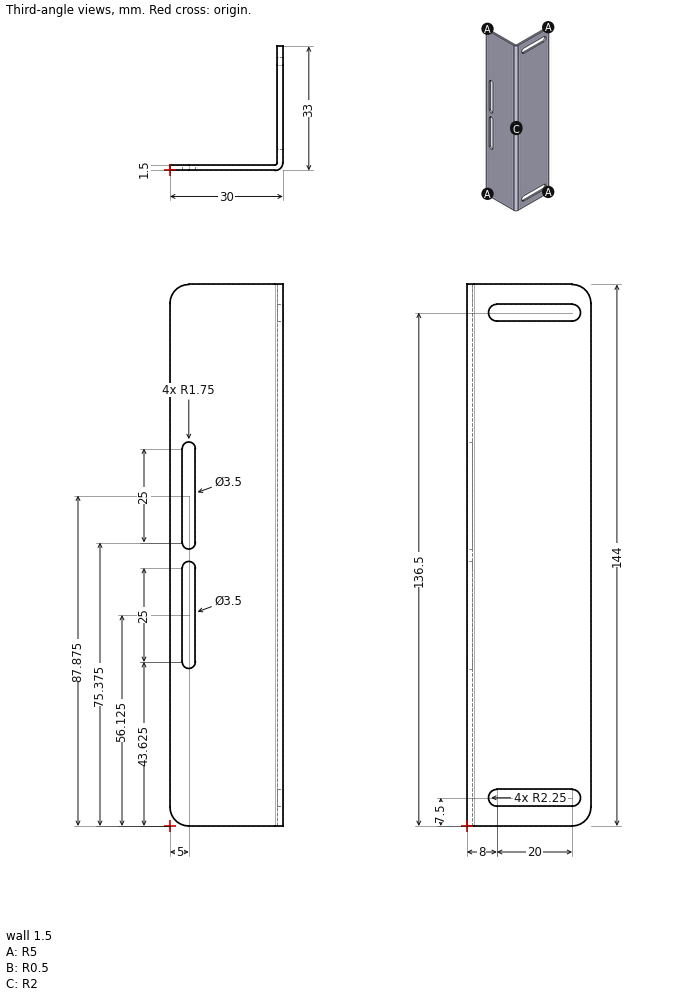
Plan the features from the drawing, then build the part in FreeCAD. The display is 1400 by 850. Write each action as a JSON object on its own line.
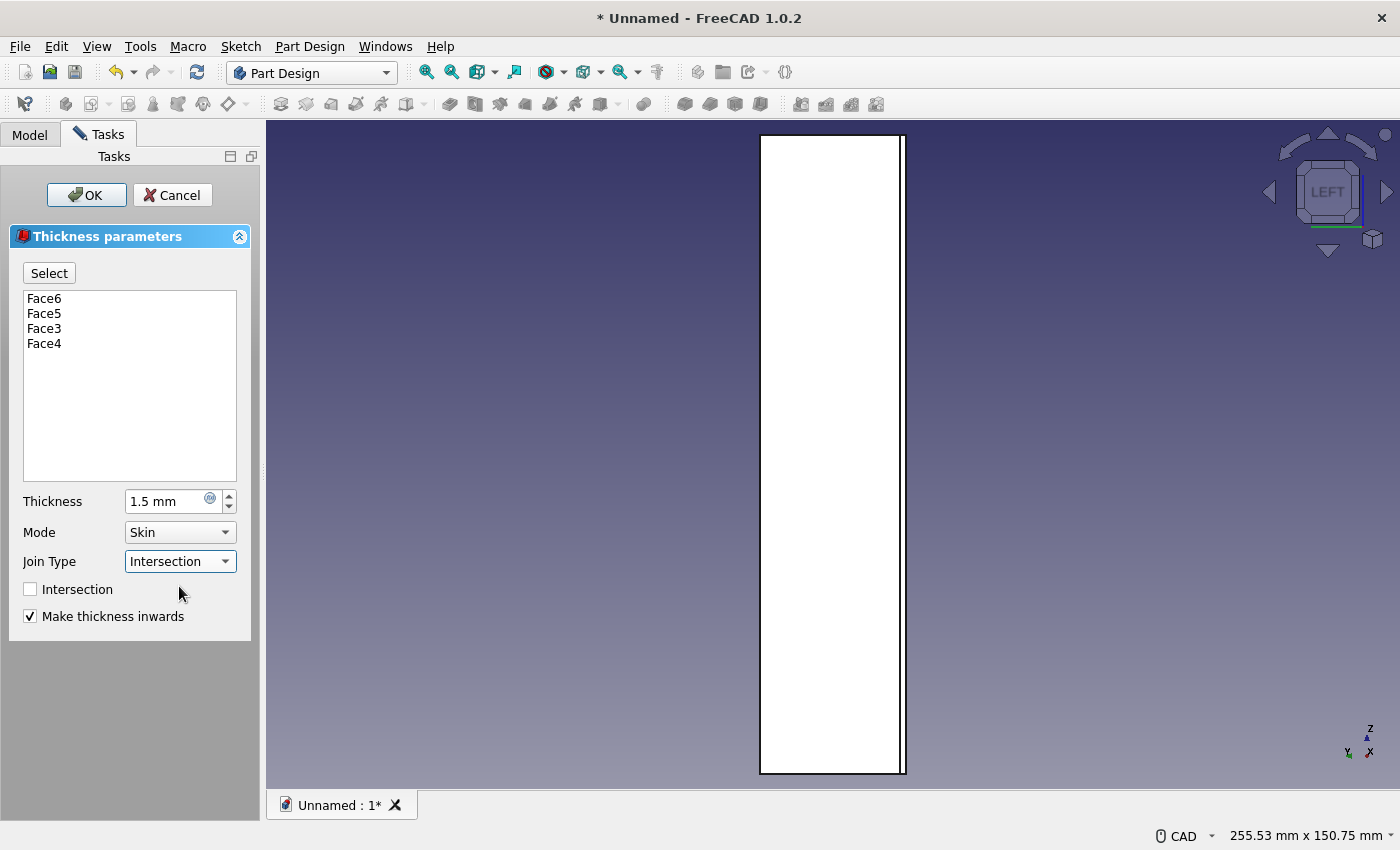
{"action": "left_click", "coordinate": [87, 195]}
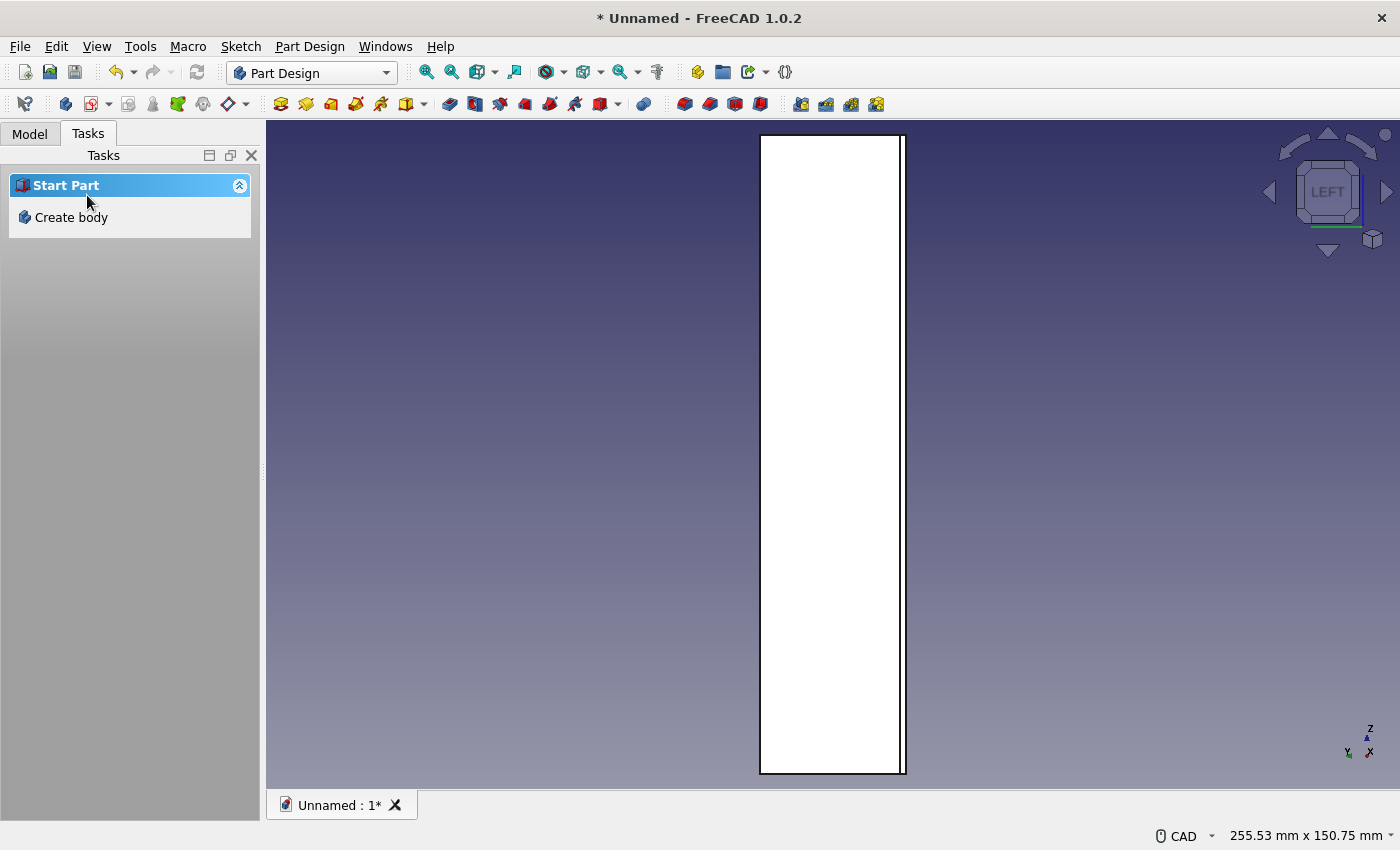
{"action": "key", "text": "0"}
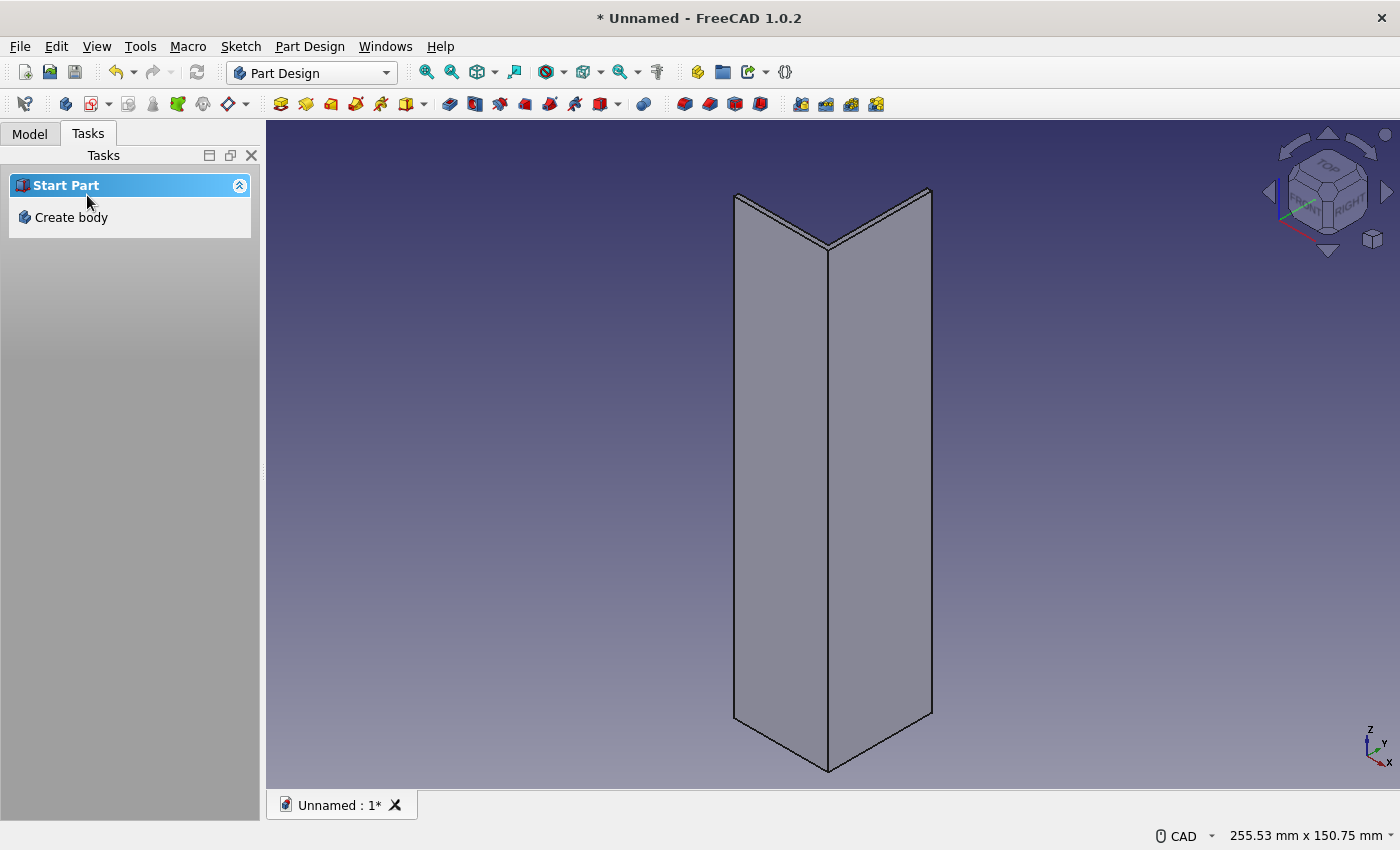
{"action": "scroll", "coordinate": [929, 189], "scroll_direction": "up", "scroll_amount": 9}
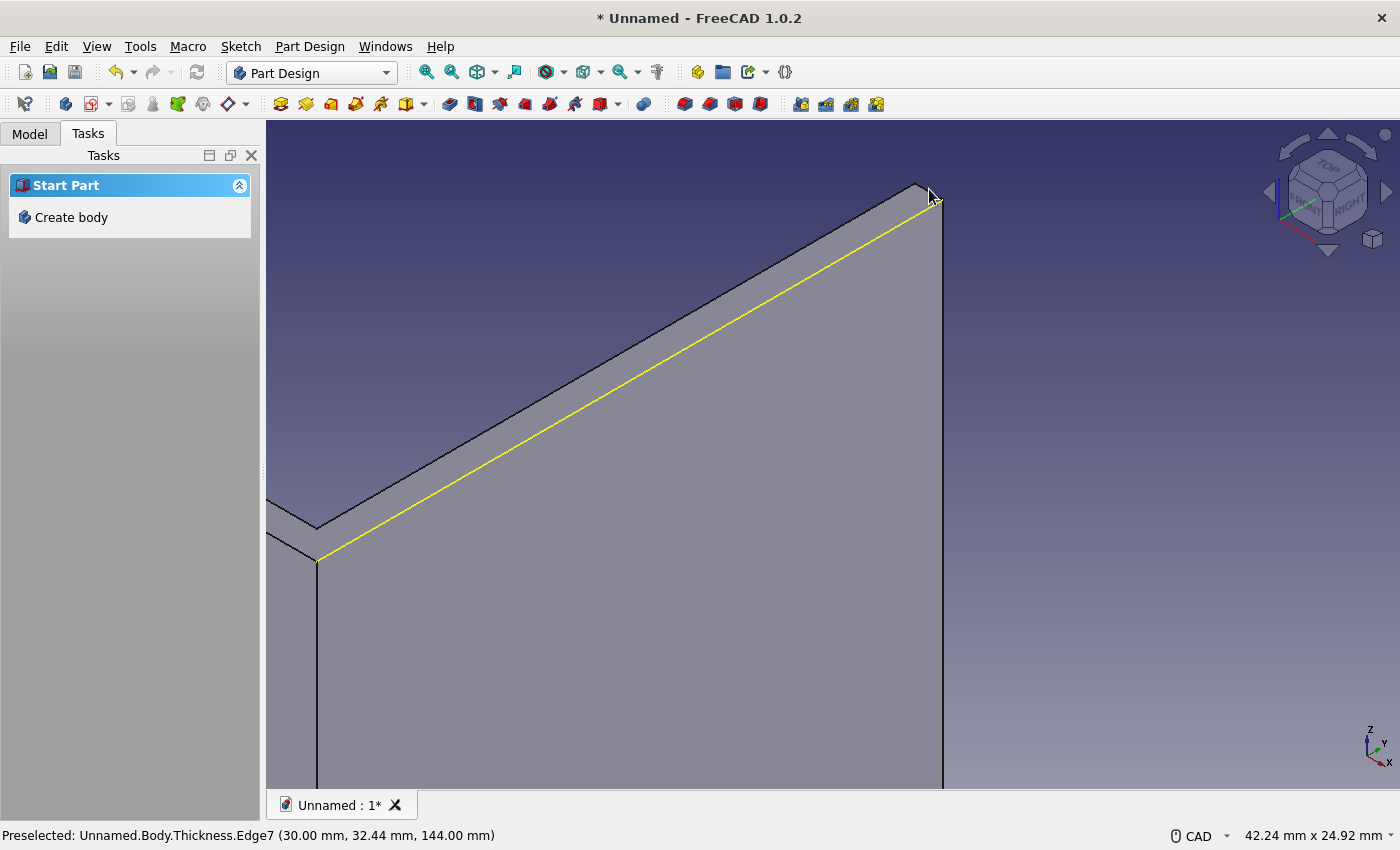
{"action": "left_click", "coordinate": [427, 72]}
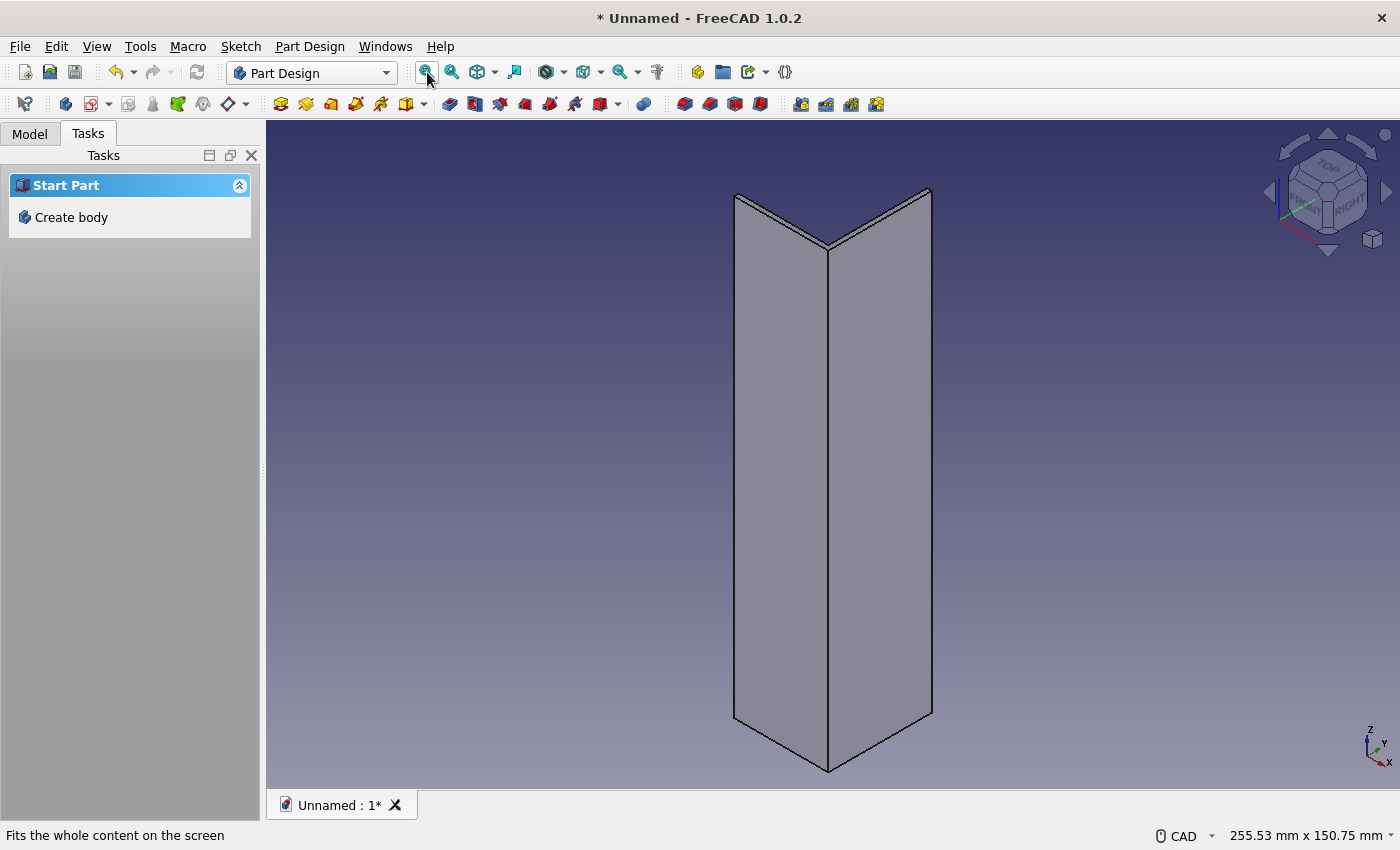
{"action": "key", "text": "2"}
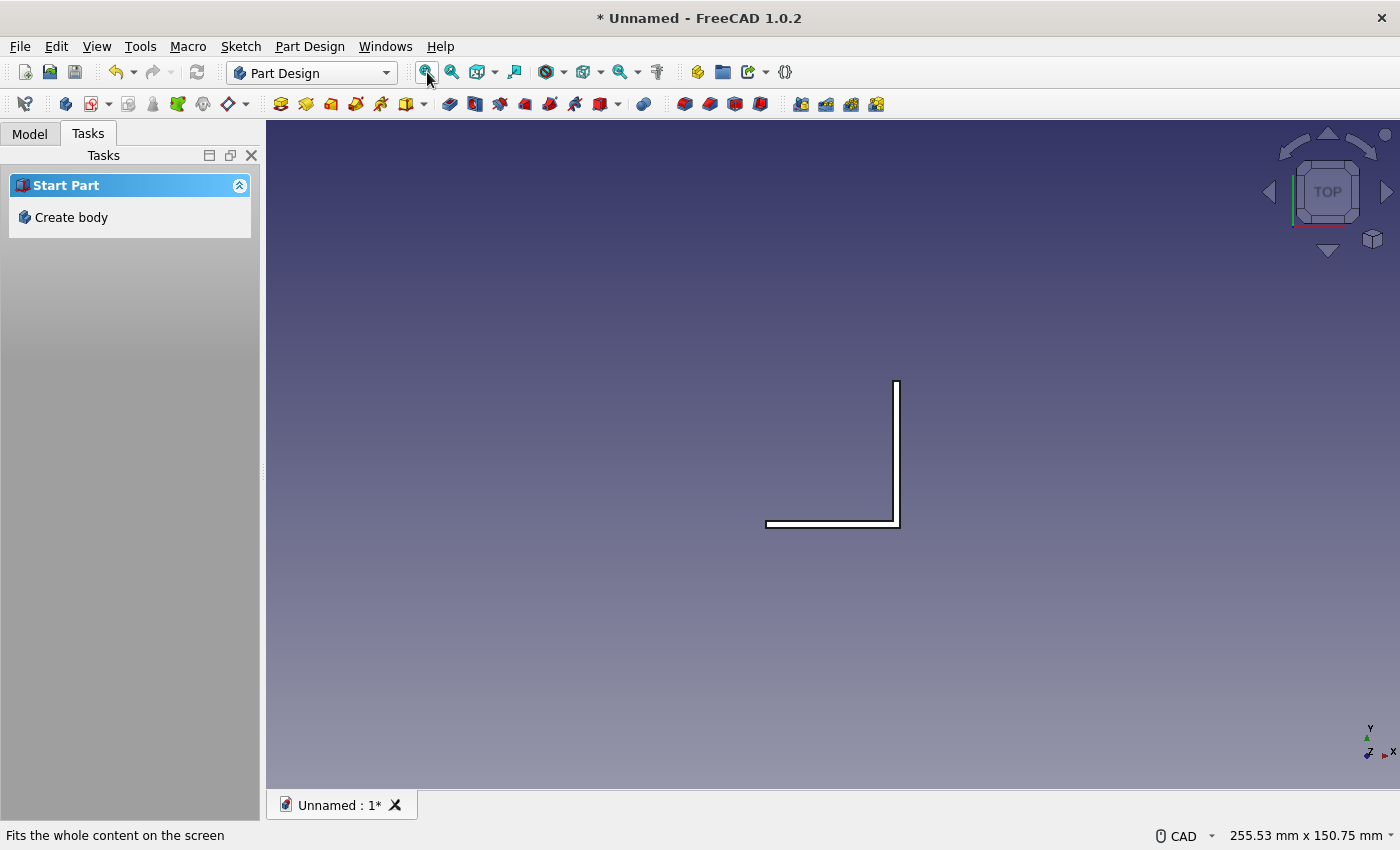
{"action": "left_click", "coordinate": [427, 72]}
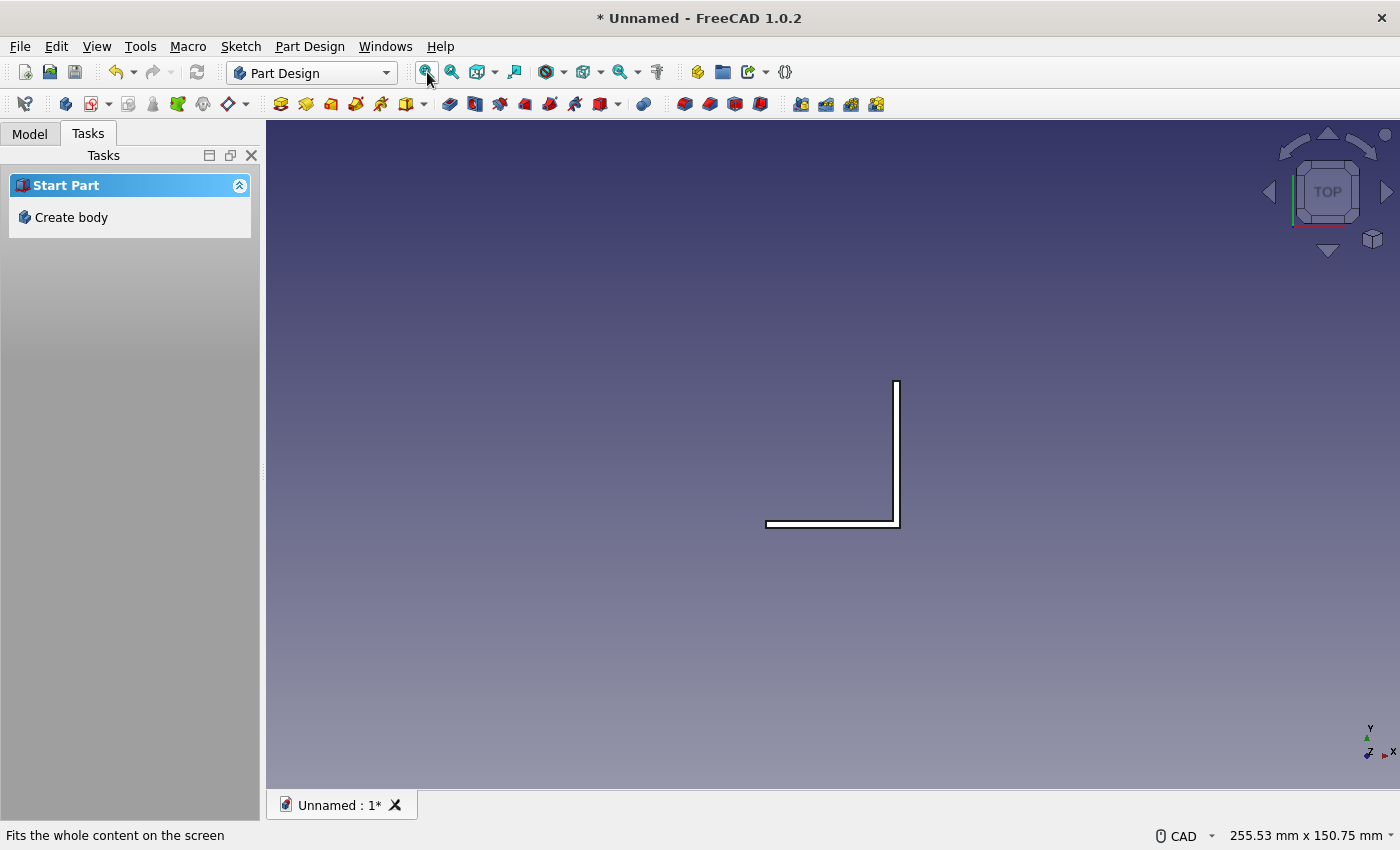
{"action": "scroll", "coordinate": [896, 380], "scroll_direction": "up", "scroll_amount": 9}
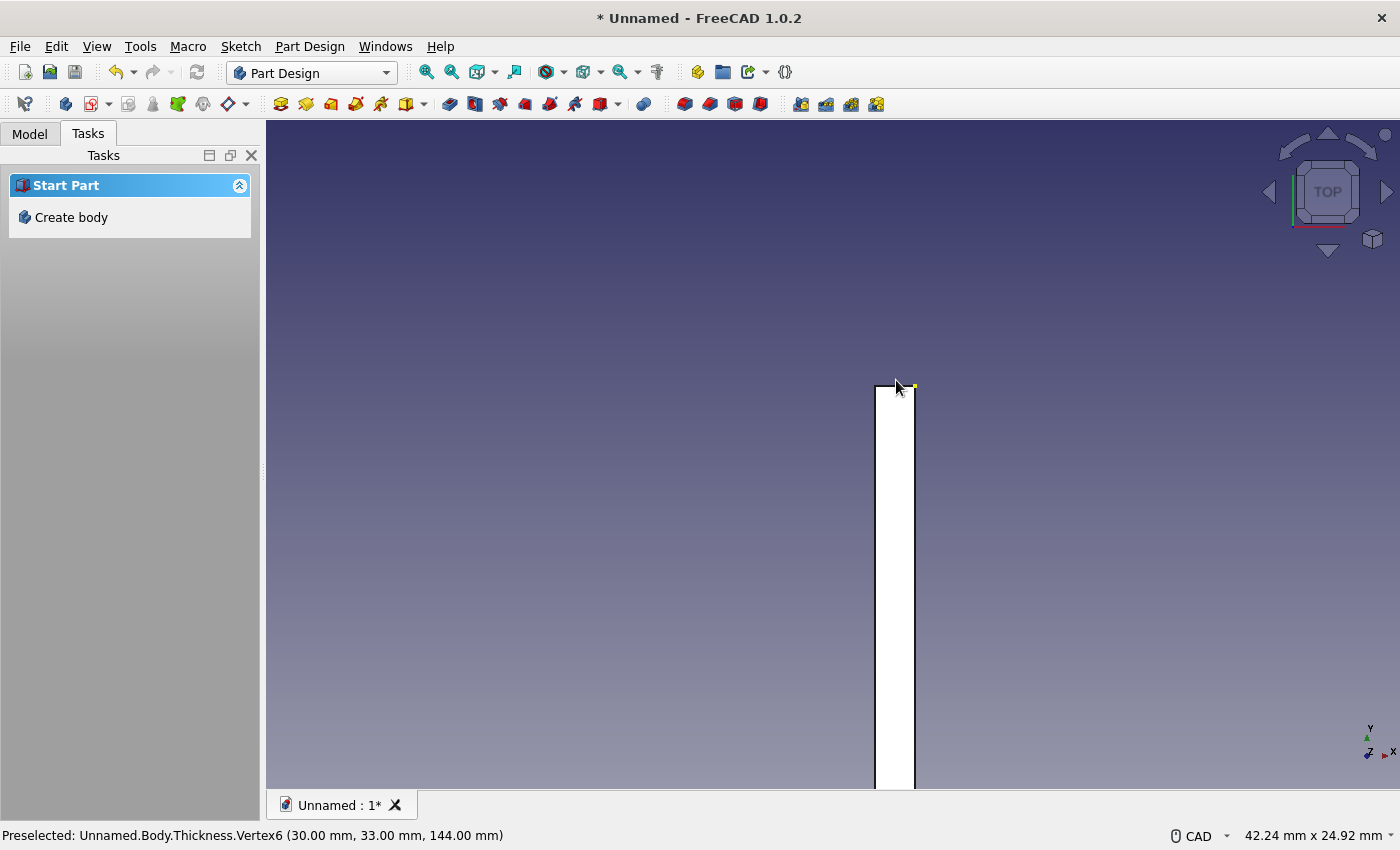
{"action": "left_click", "coordinate": [895, 385]}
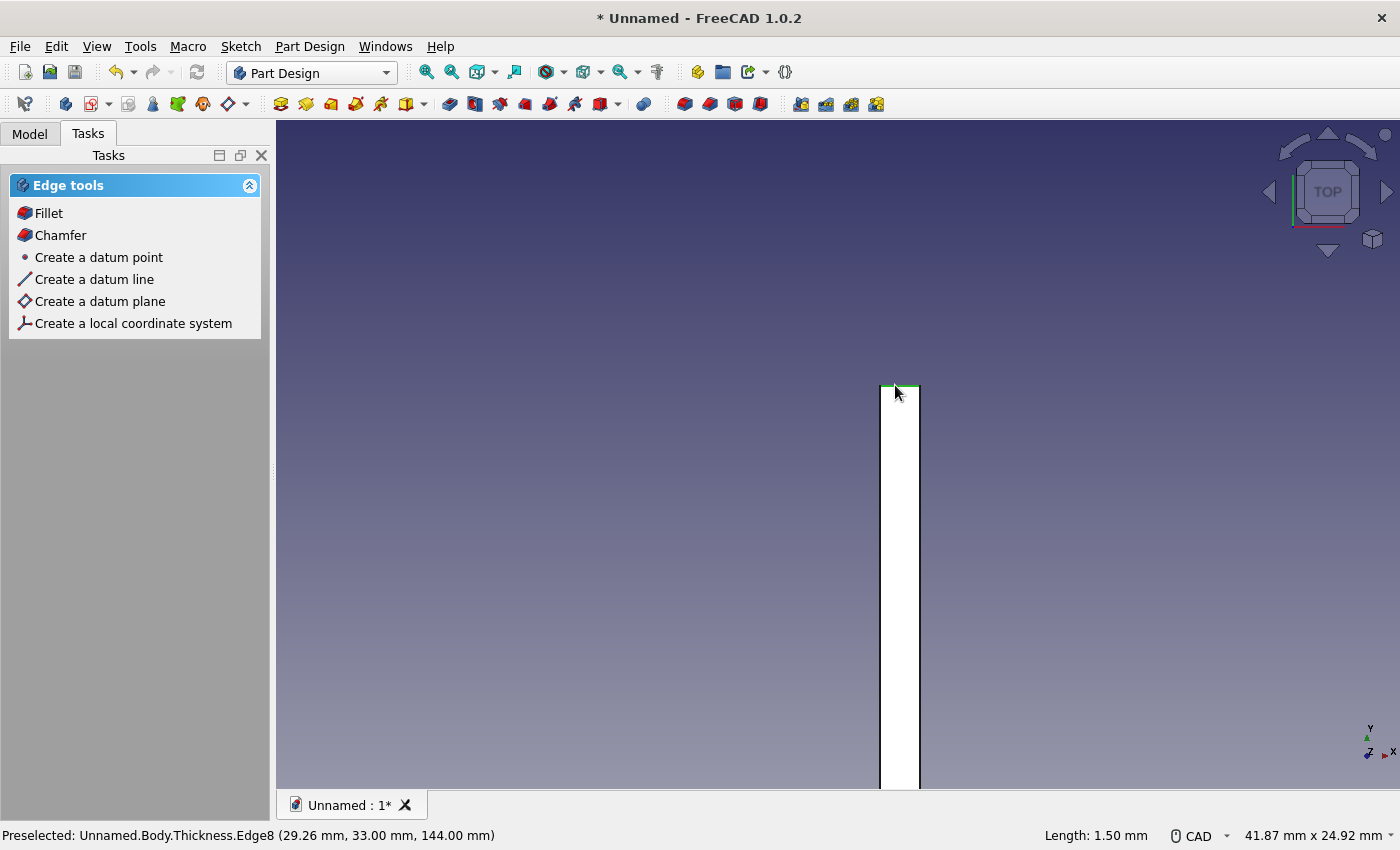
{"action": "left_click", "coordinate": [427, 72]}